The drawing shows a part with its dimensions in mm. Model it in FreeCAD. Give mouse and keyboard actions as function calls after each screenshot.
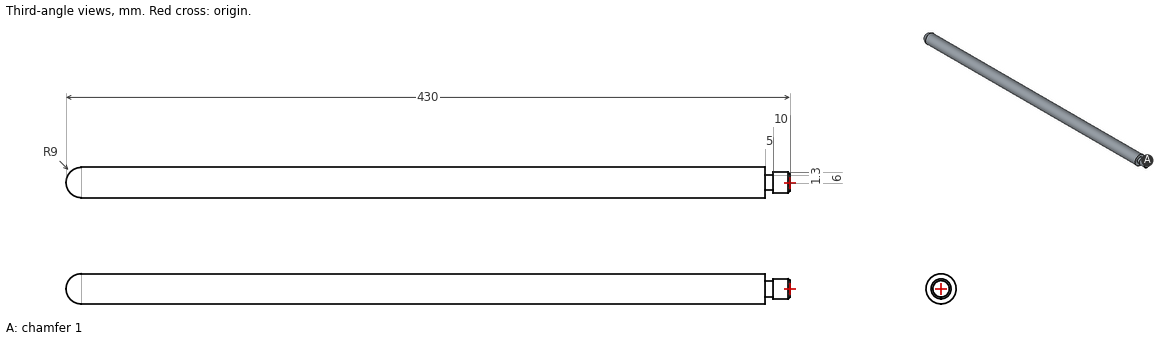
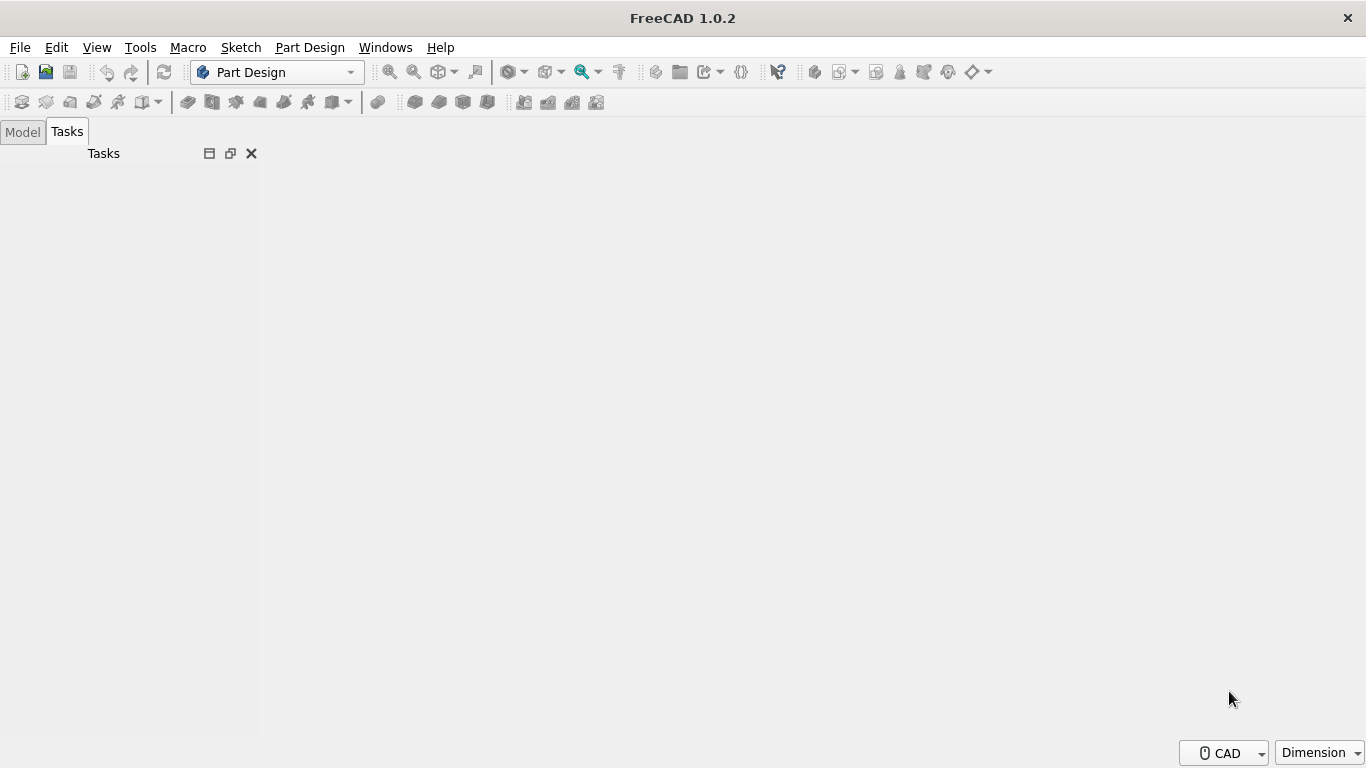
click(22, 72)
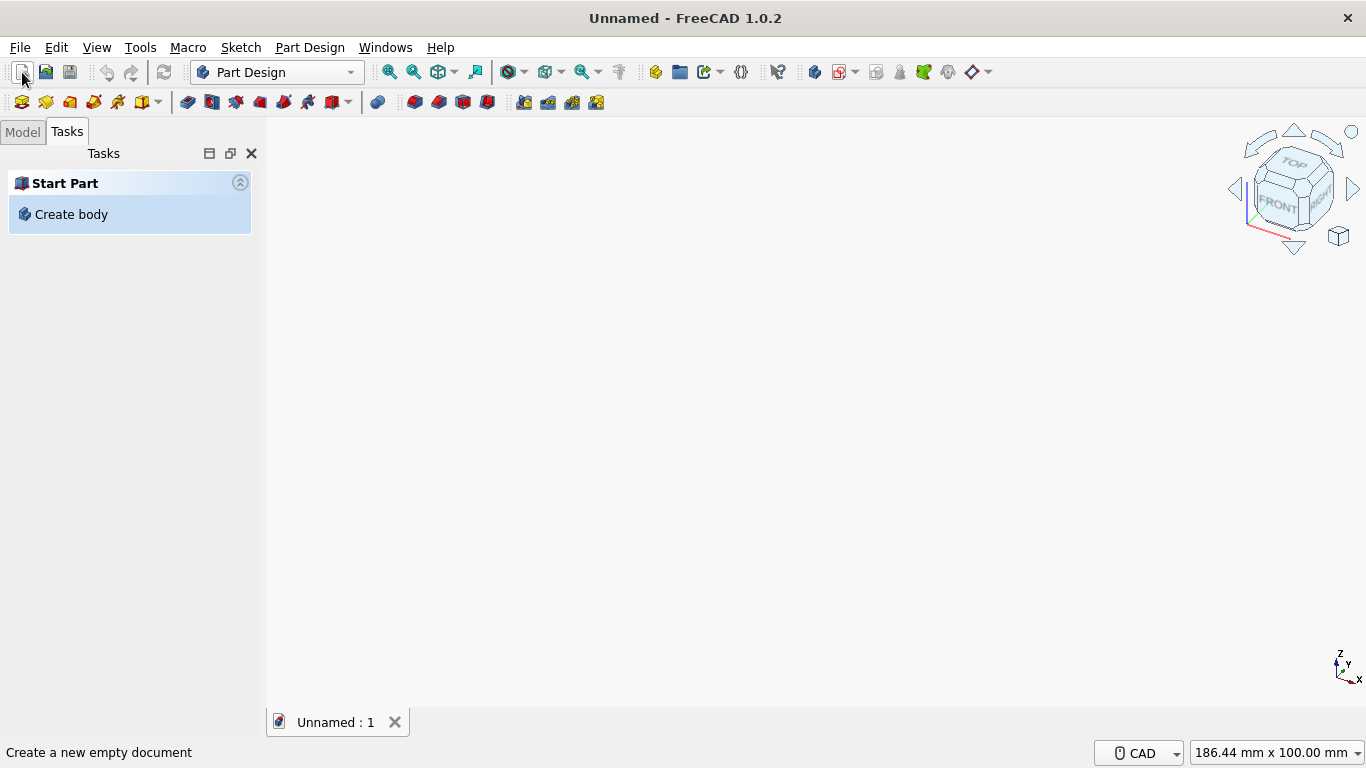
click(840, 72)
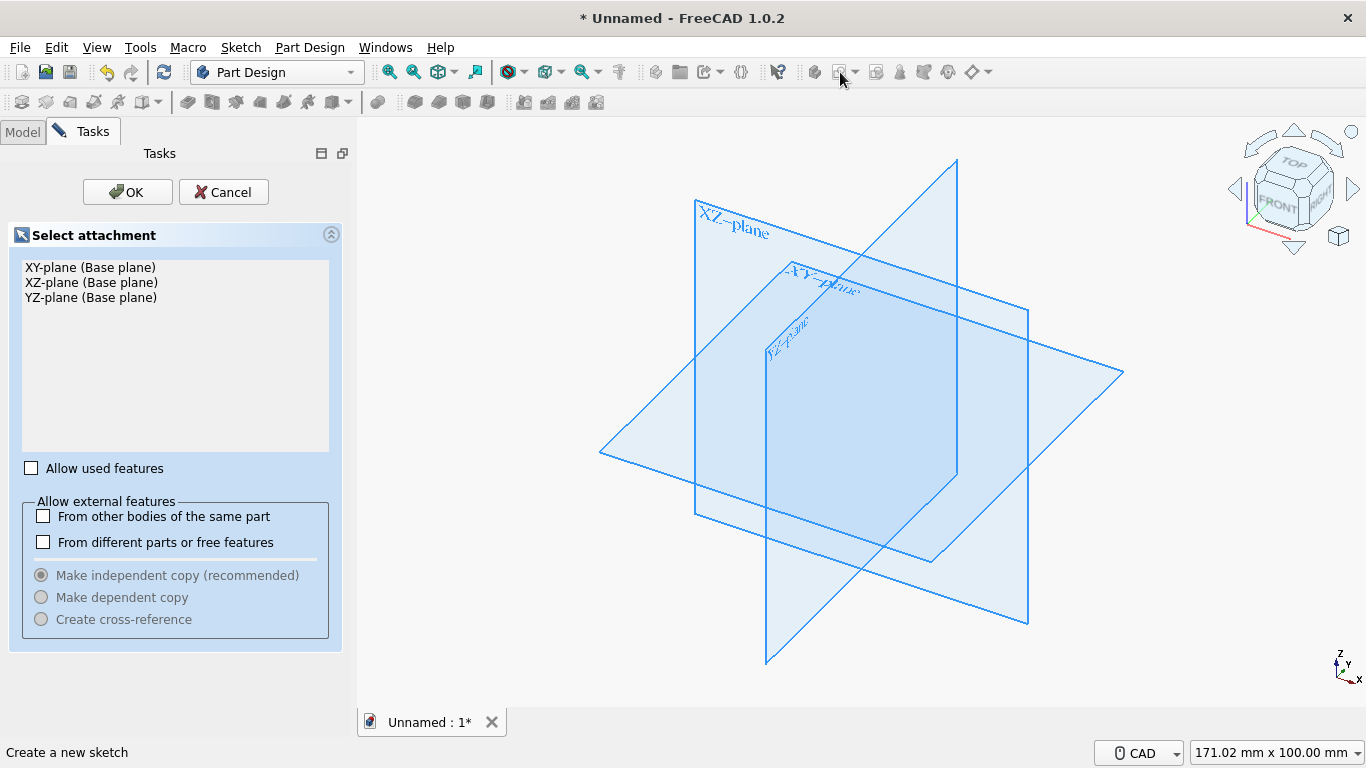
click(82, 268)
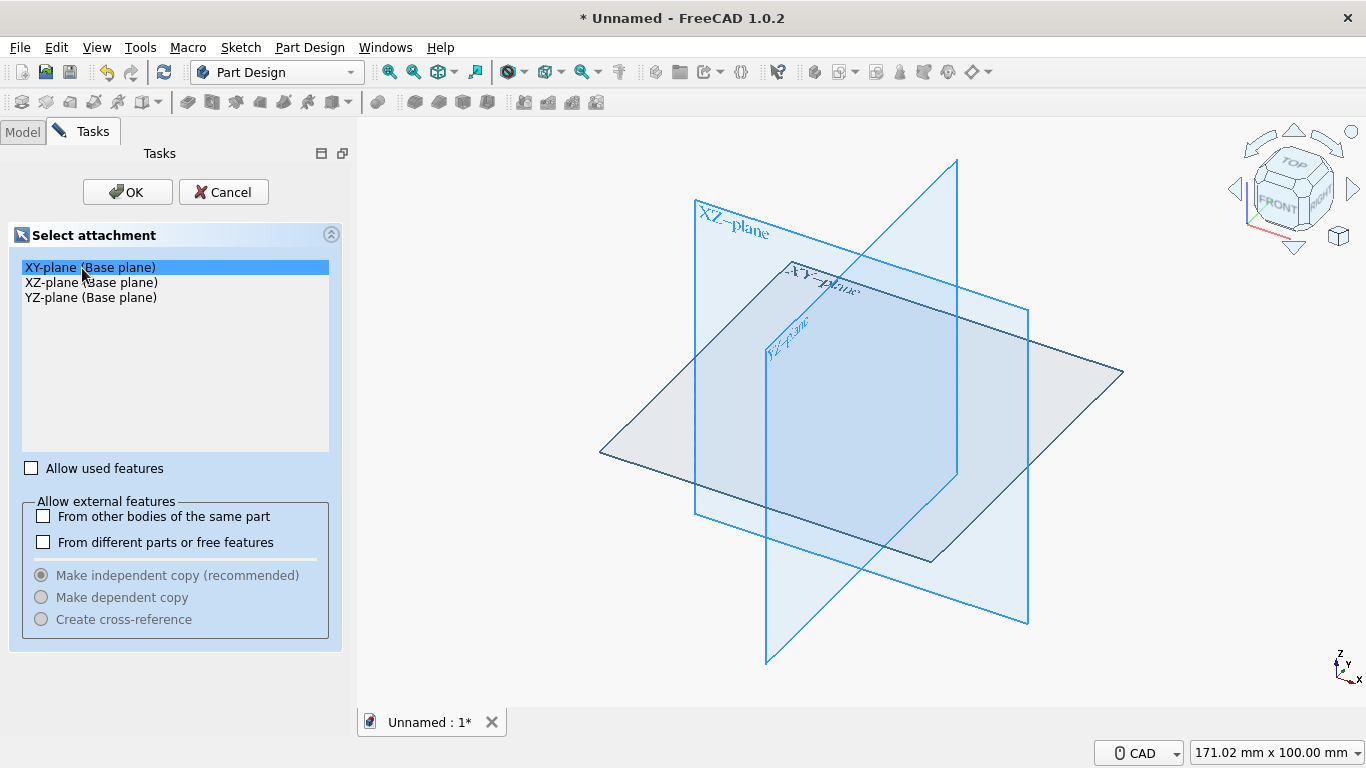
click(128, 192)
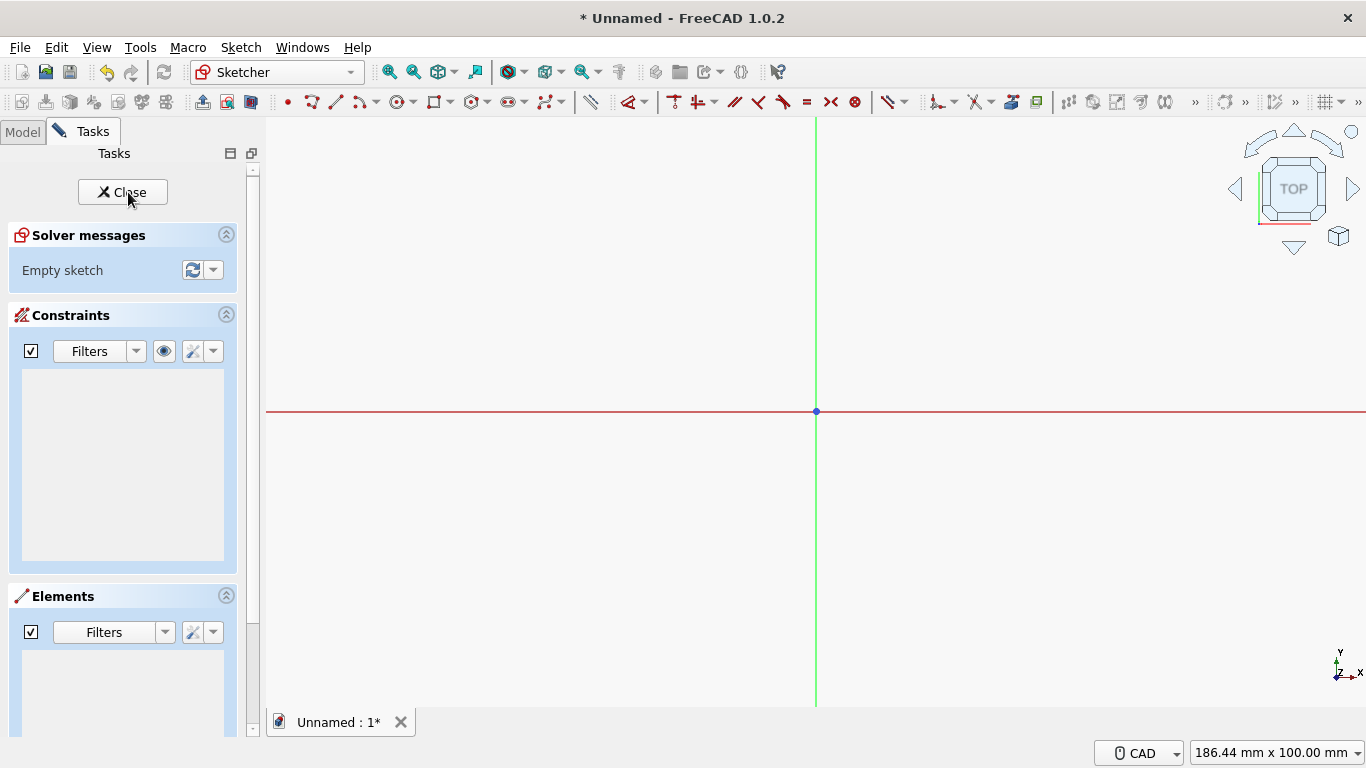
scroll(1140, 421, down, 7)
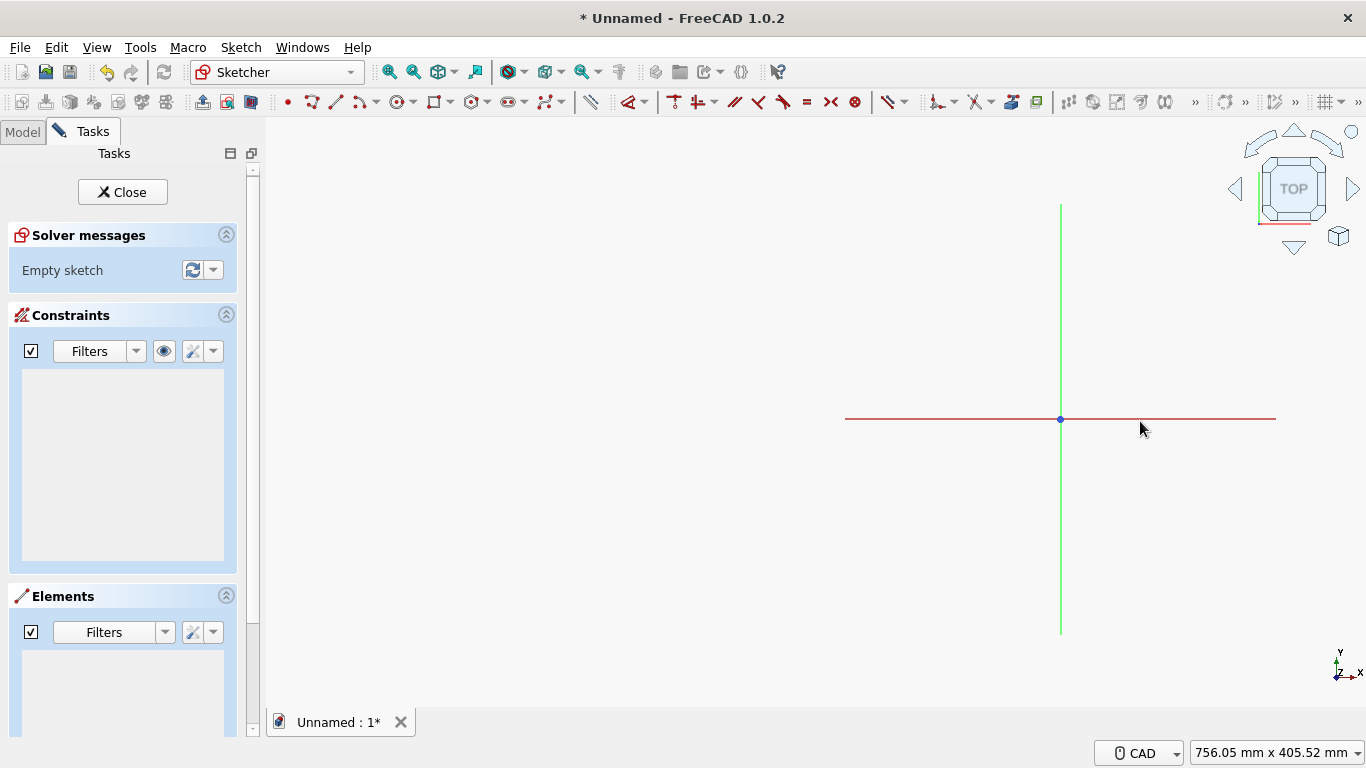
click(312, 102)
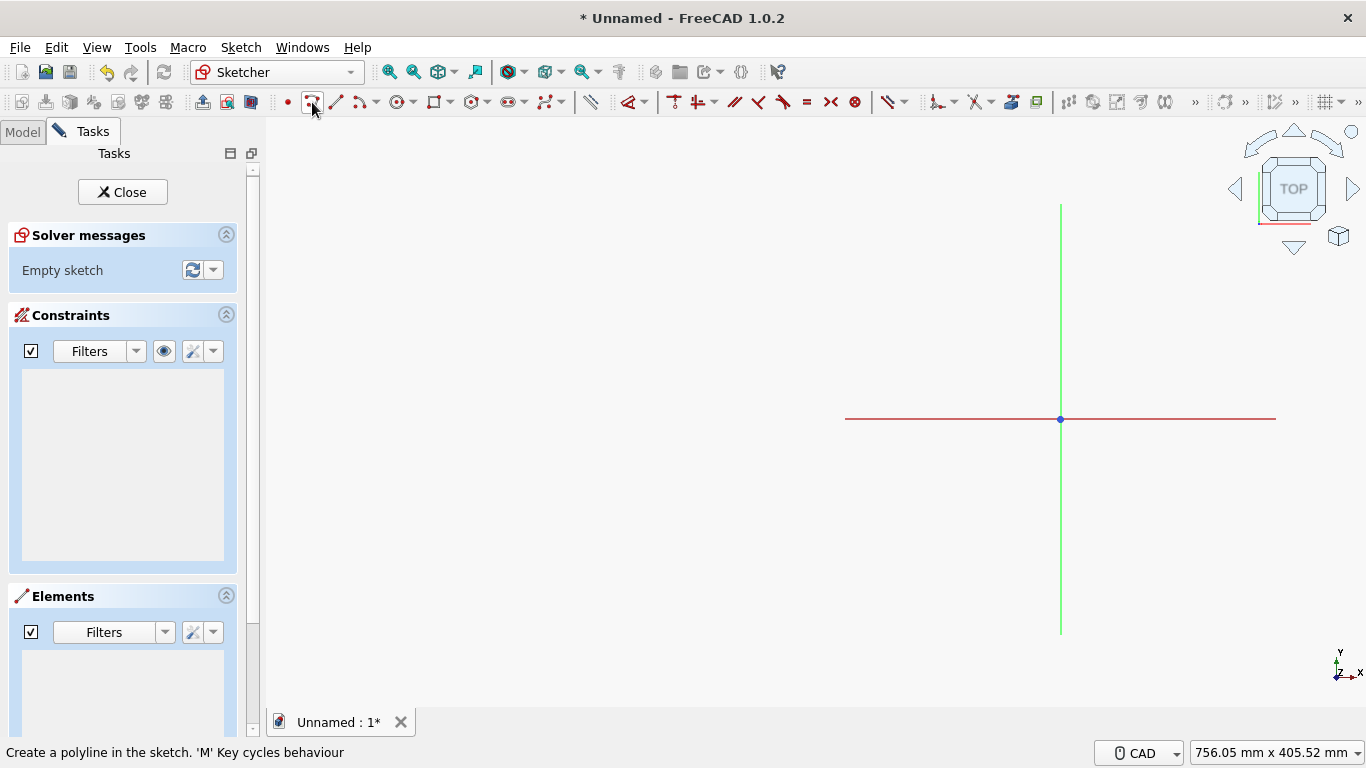
click(435, 419)
click(1061, 419)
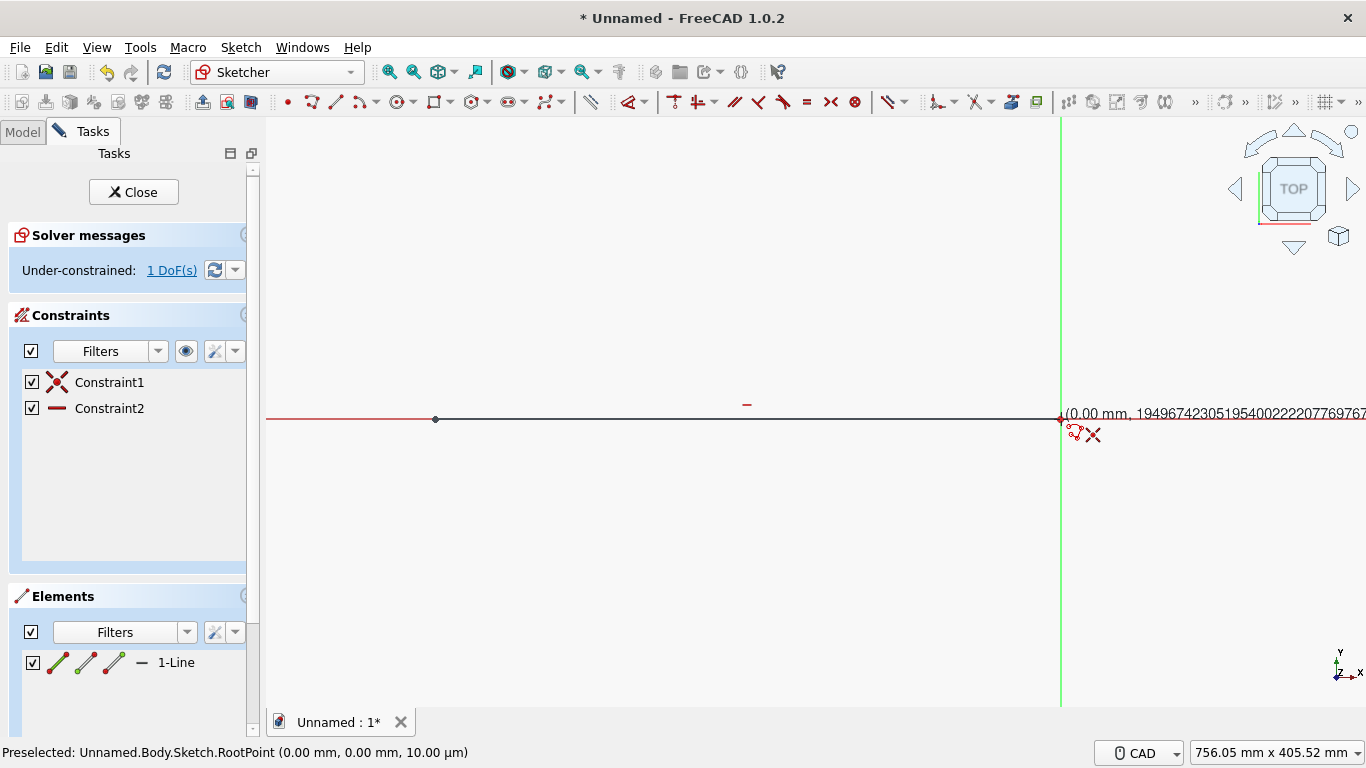
scroll(1061, 410, up, 3)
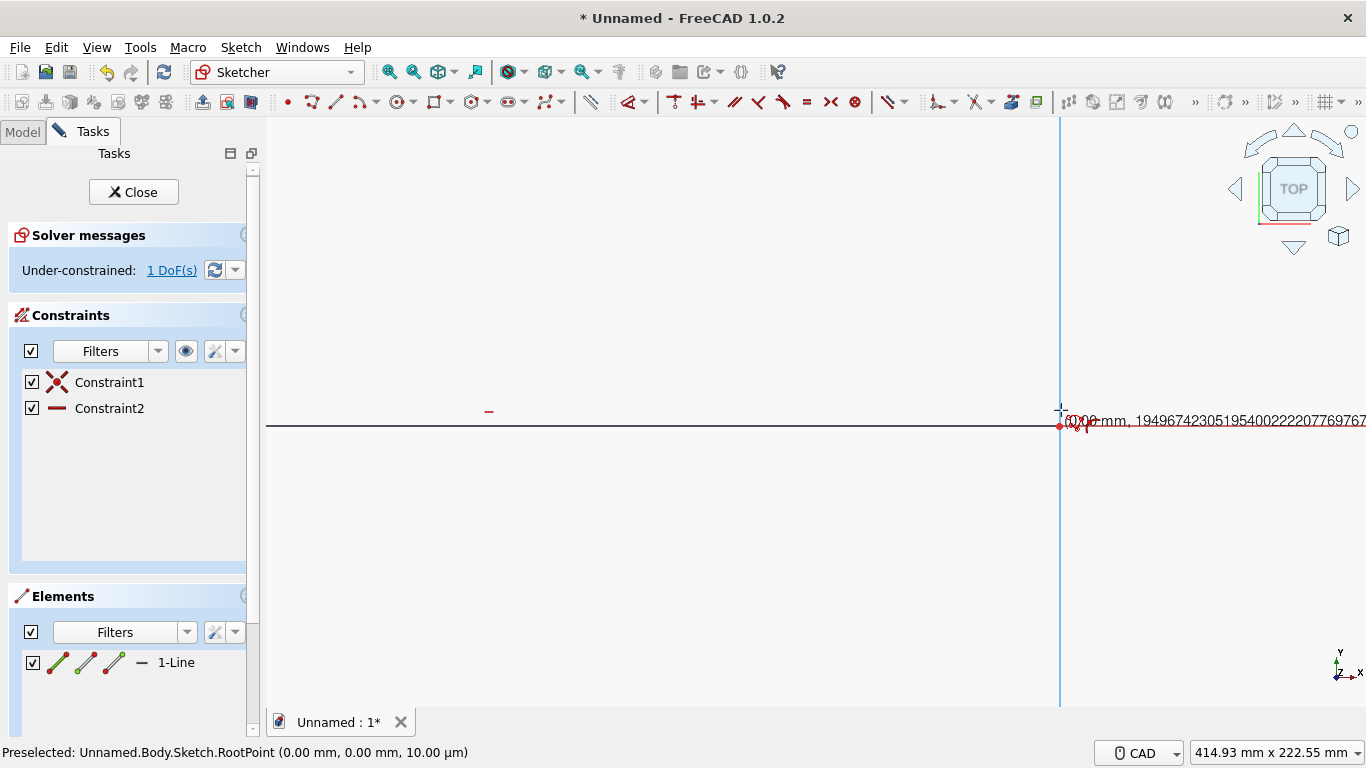
click(1051, 410)
click(1033, 410)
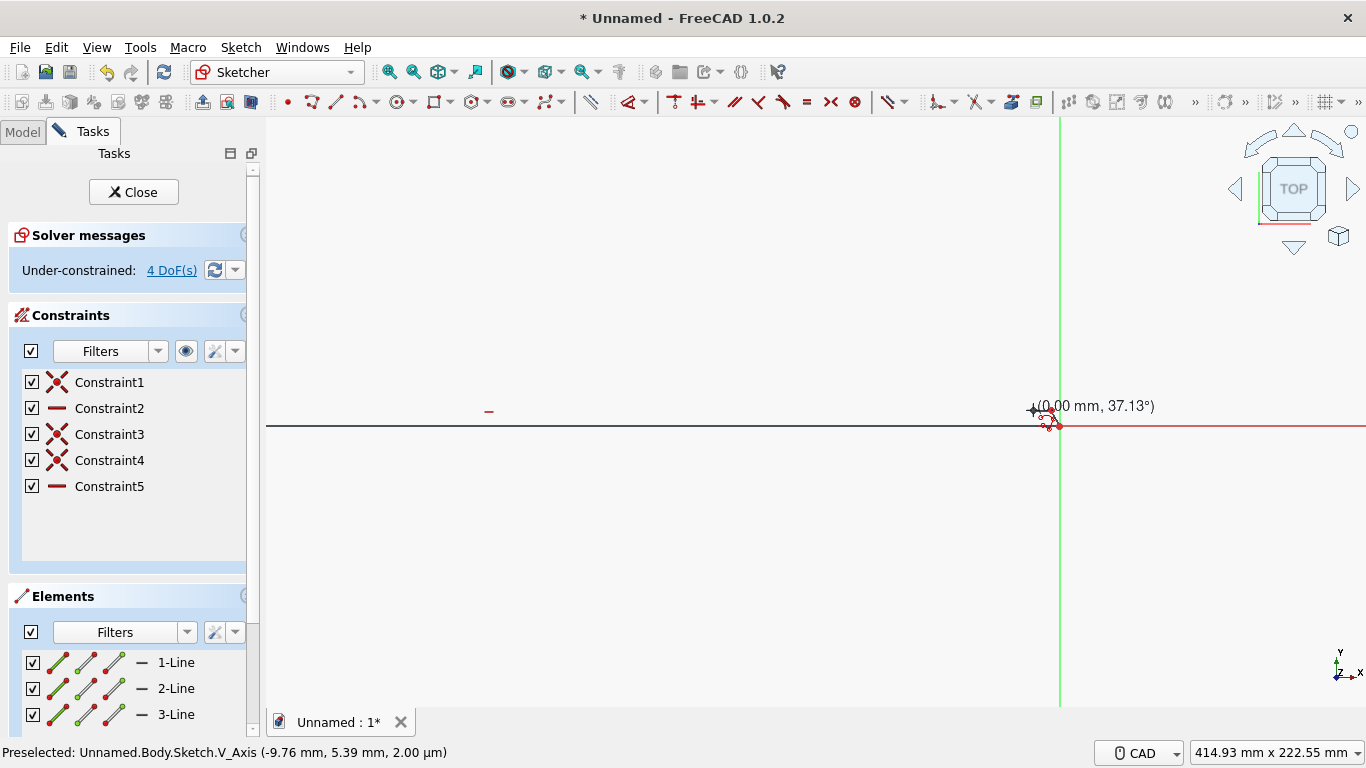
scroll(1033, 414, up, 8)